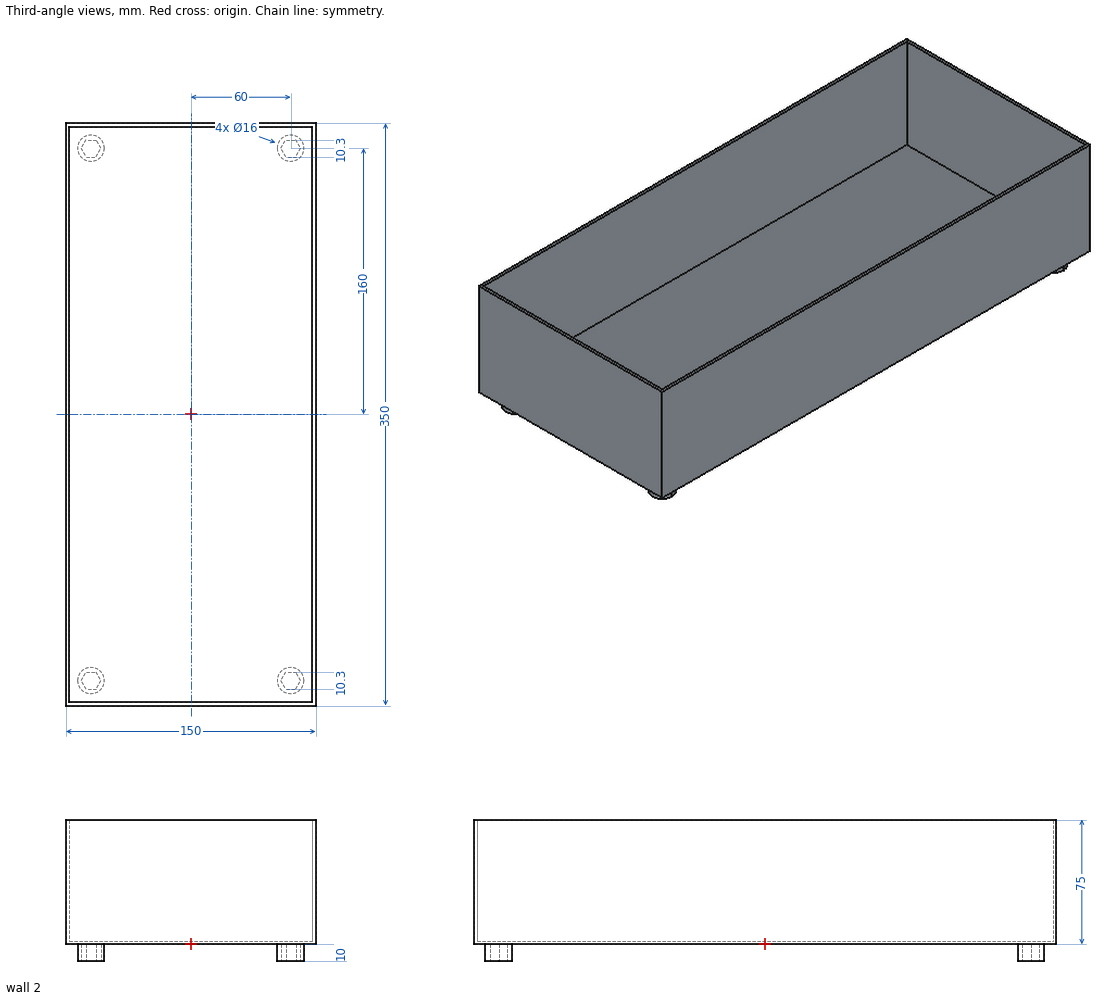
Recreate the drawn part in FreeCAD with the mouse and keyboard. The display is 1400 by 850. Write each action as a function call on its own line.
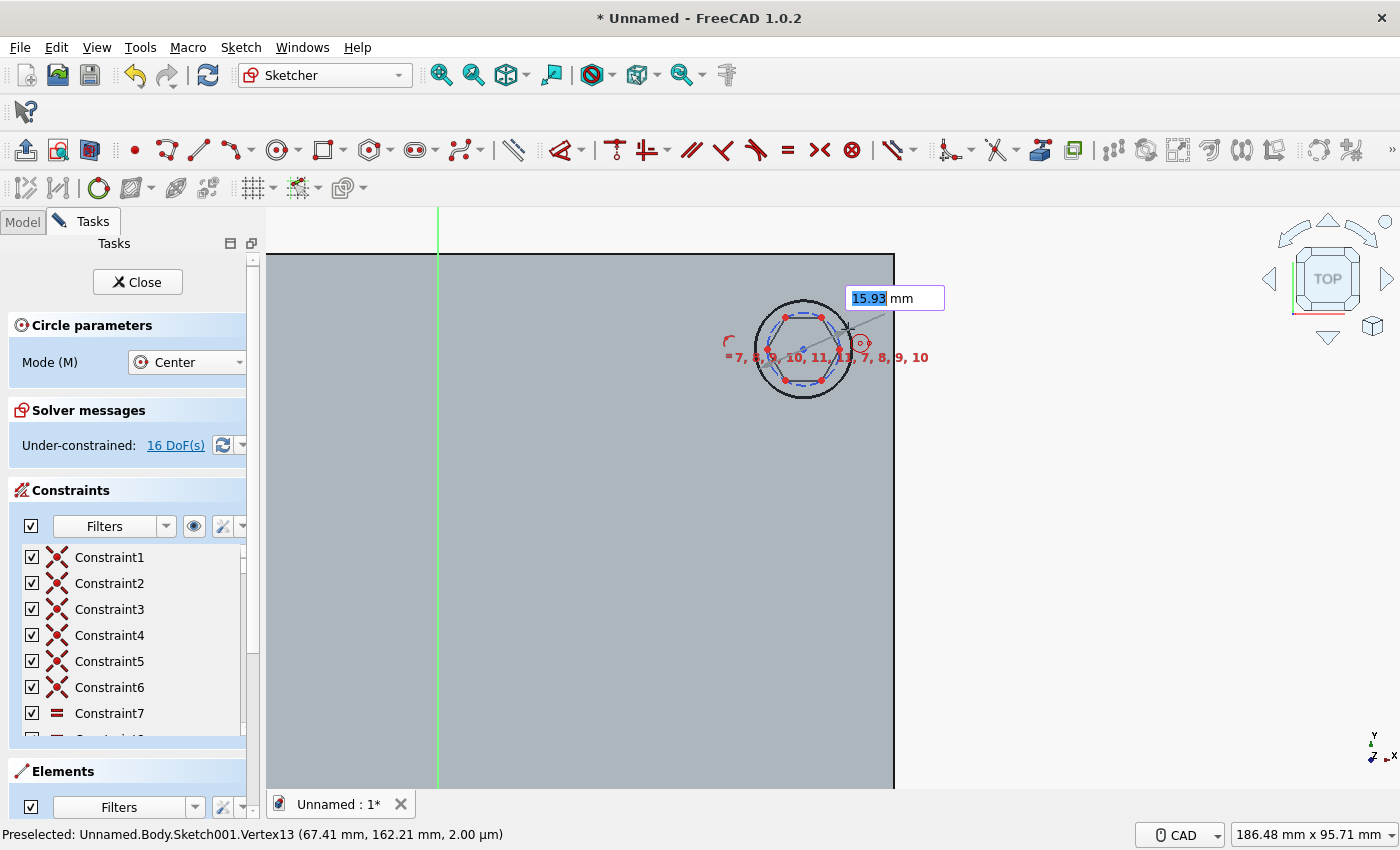
text(16)
key(Return)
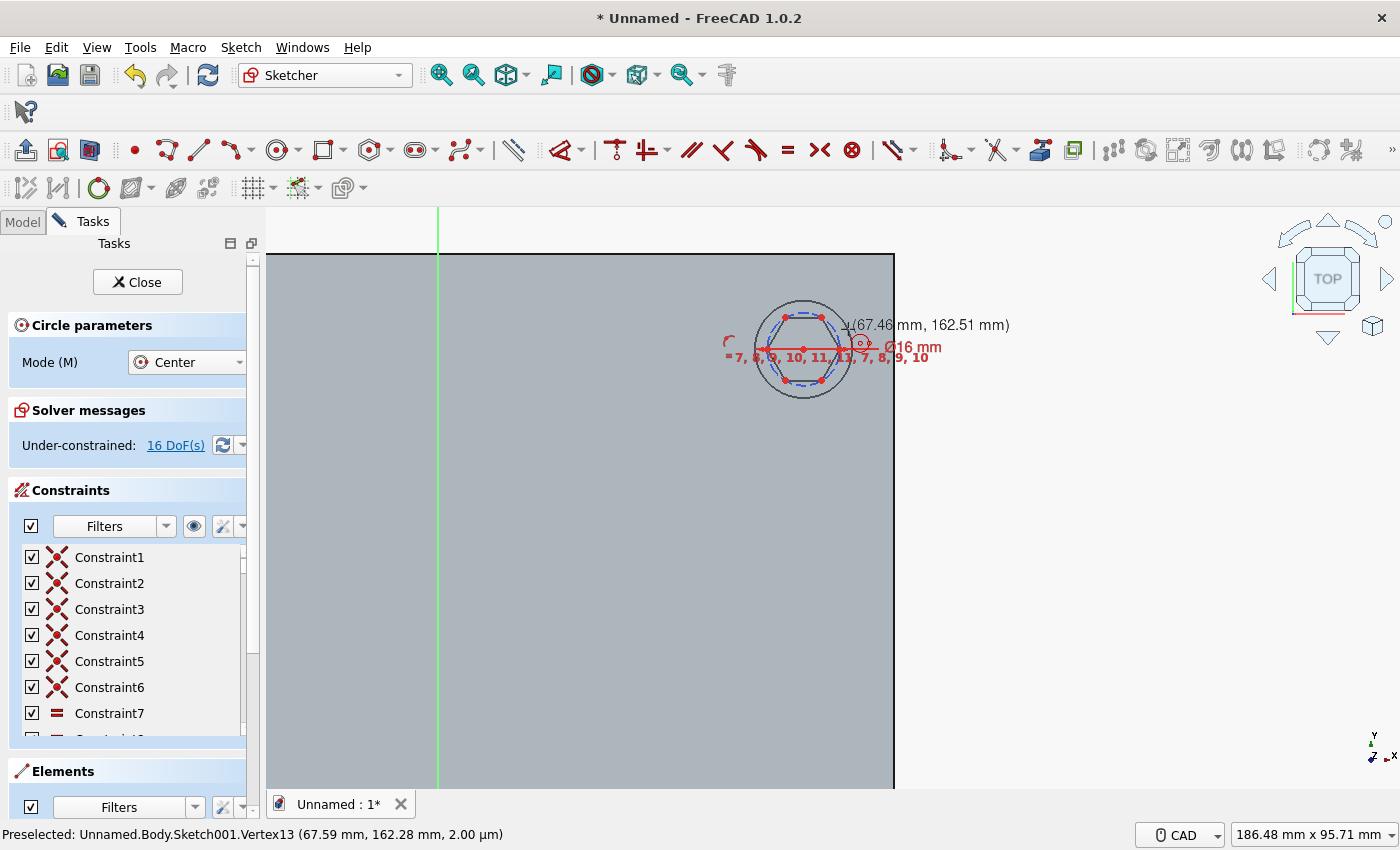
scroll(829, 336, down, 9)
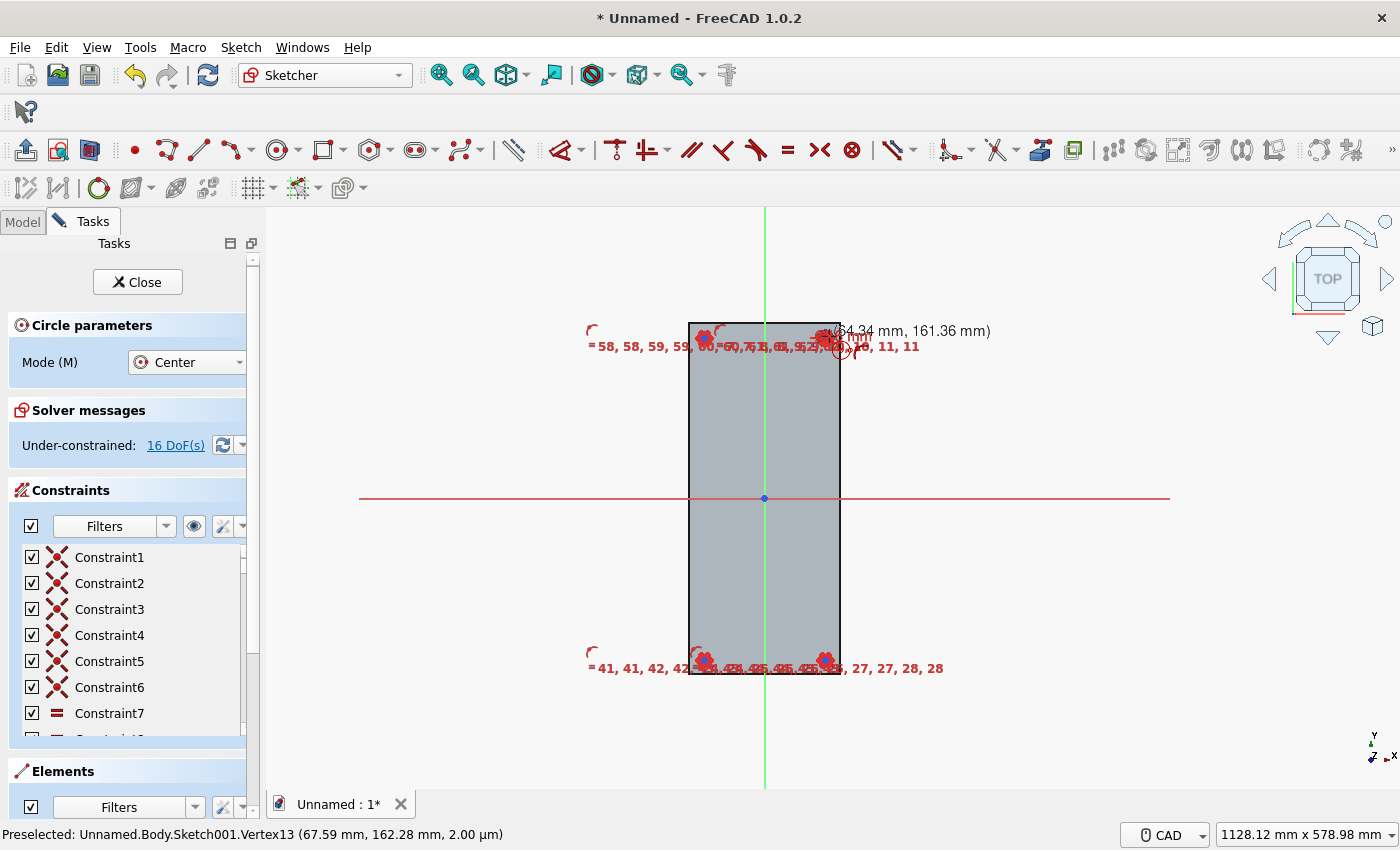
scroll(825, 659, up, 6)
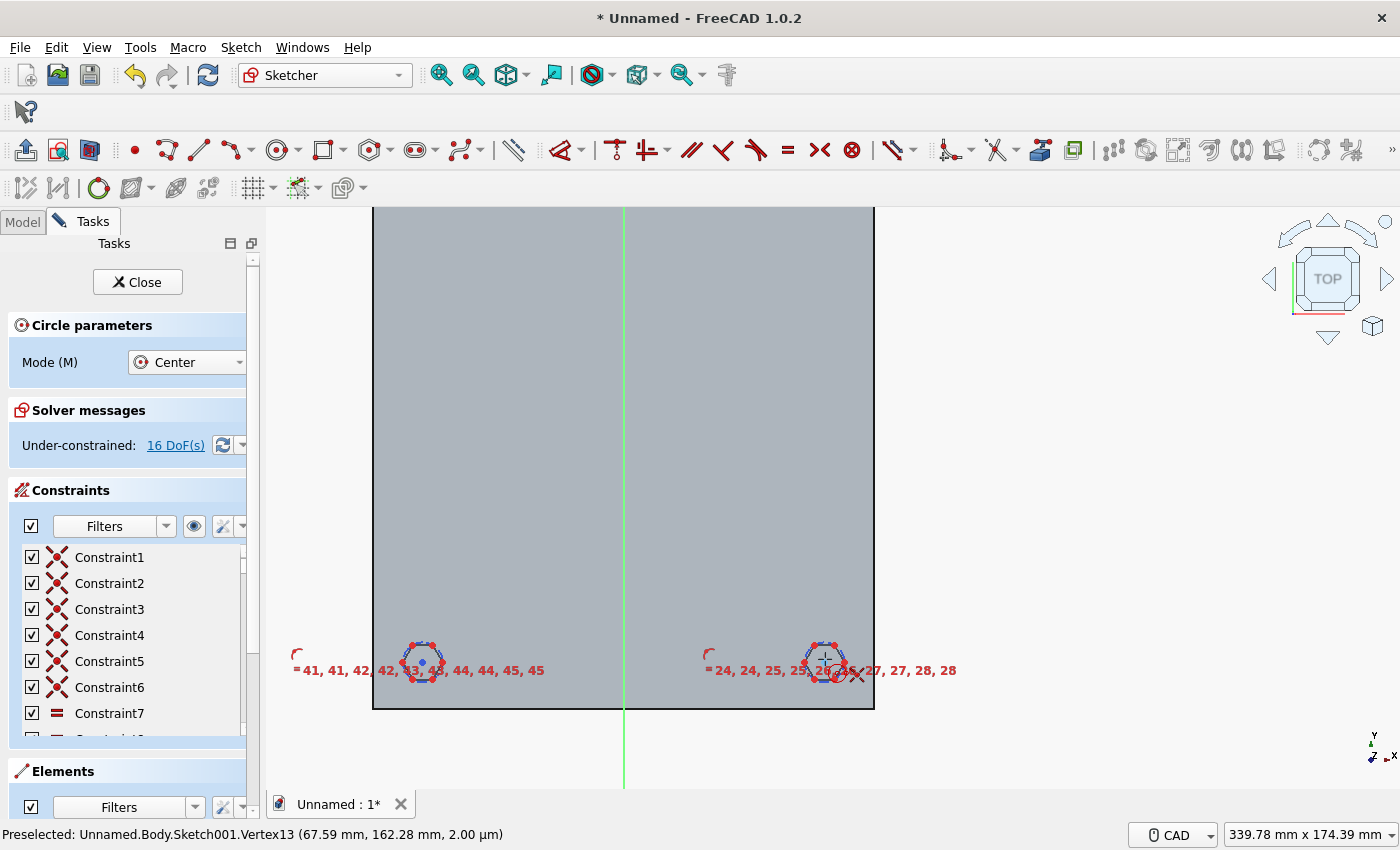
click(825, 662)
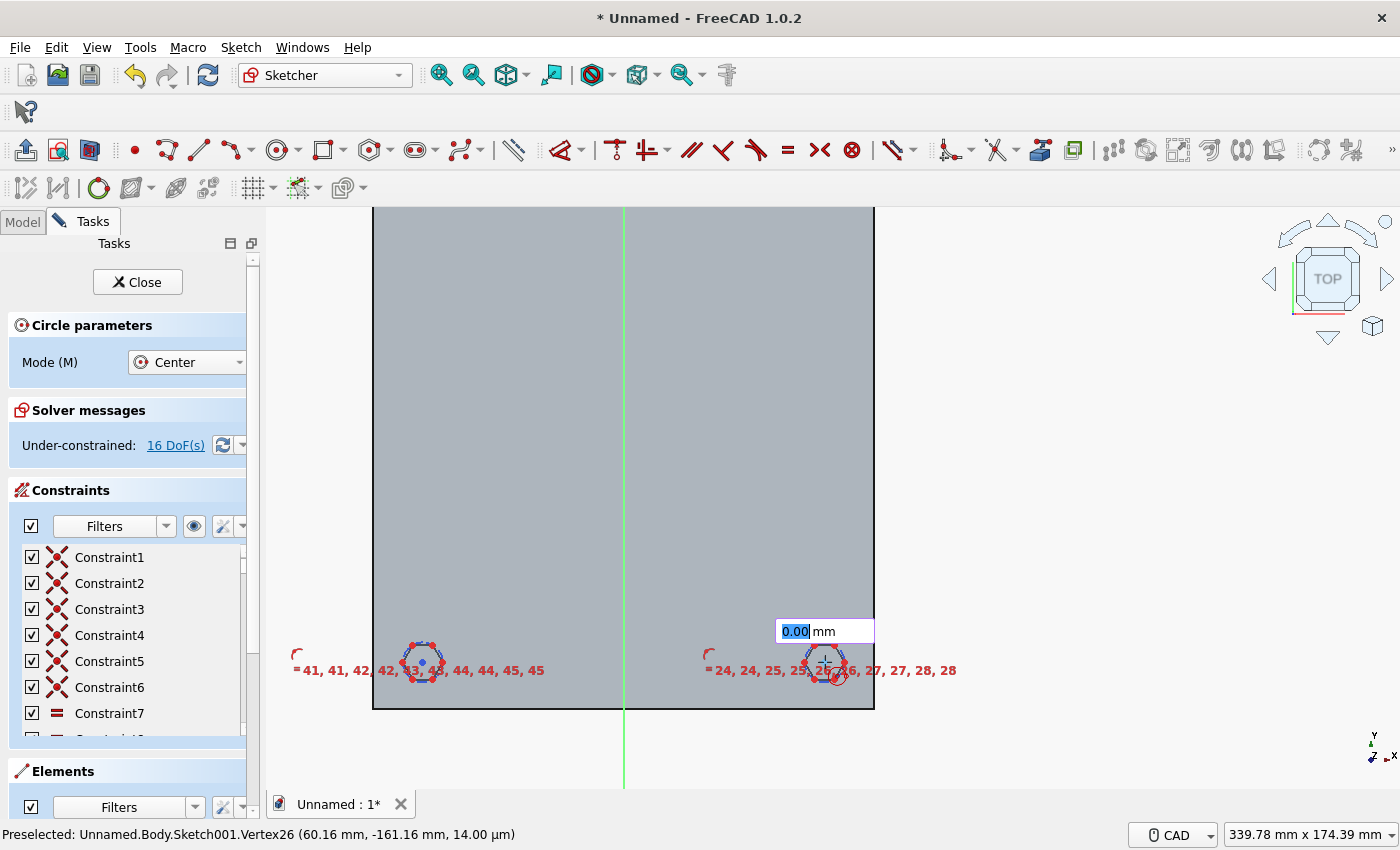
scroll(849, 649, up, 3)
move(849, 649)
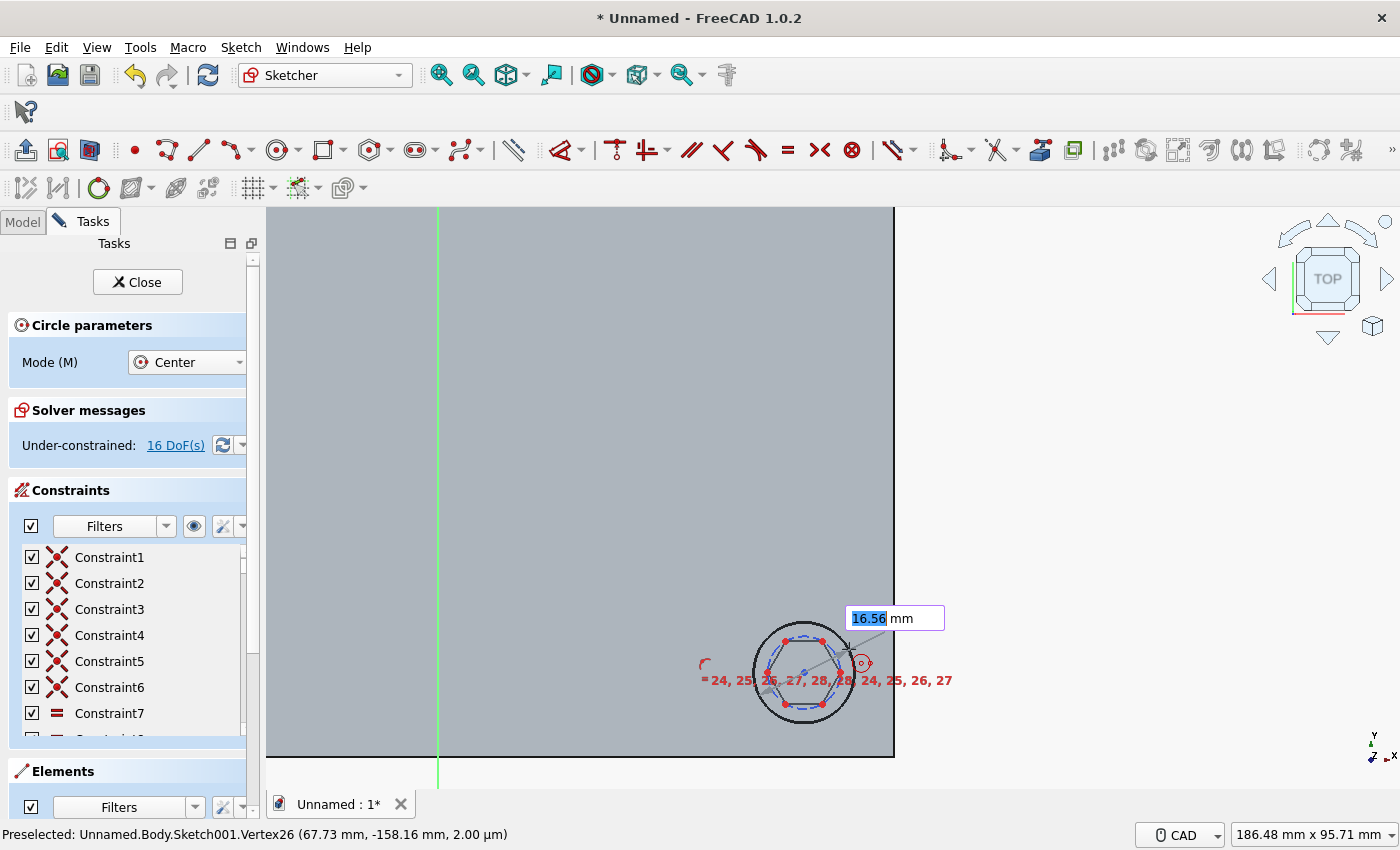
text(16)
key(Return)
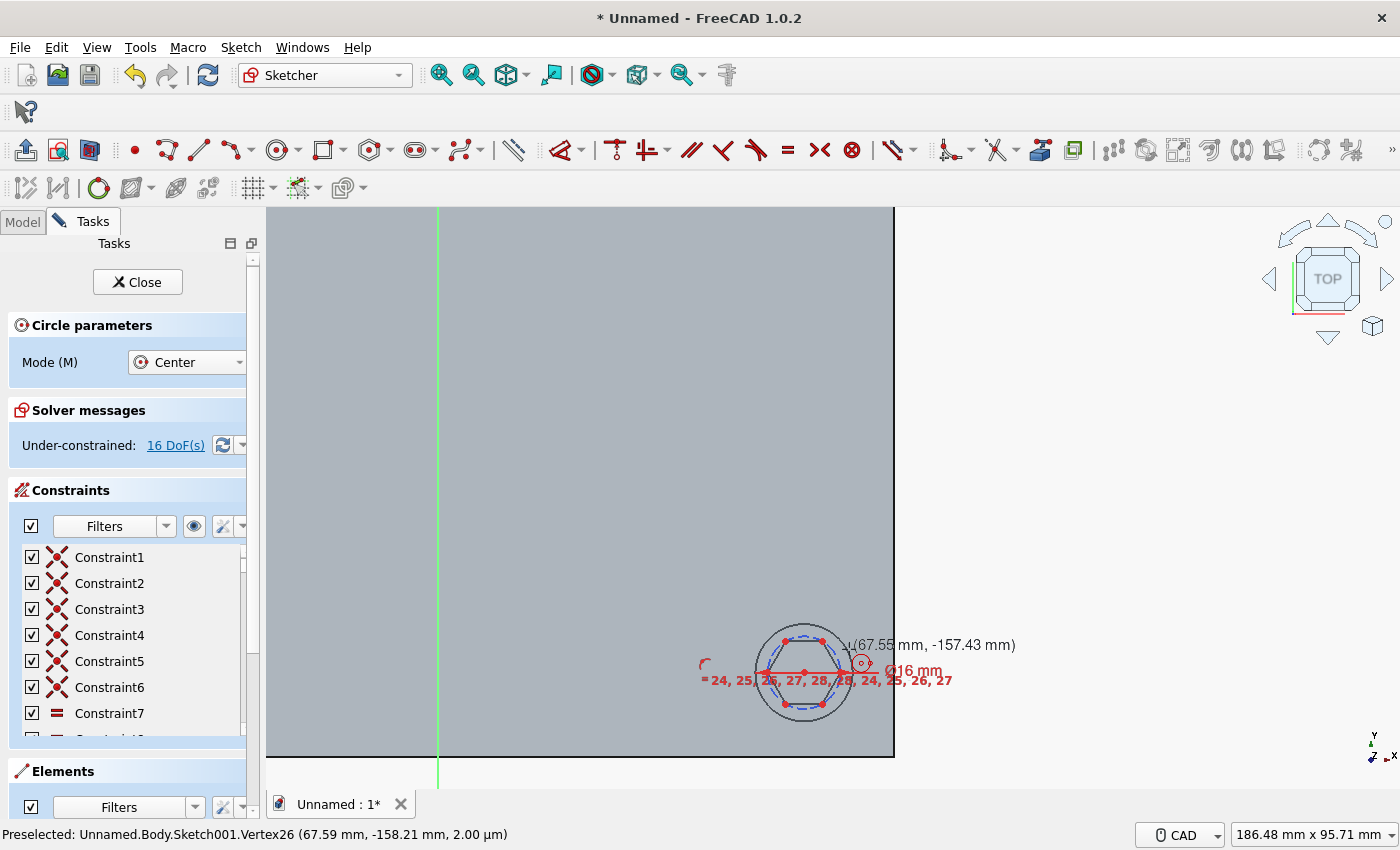
scroll(829, 657, down, 9)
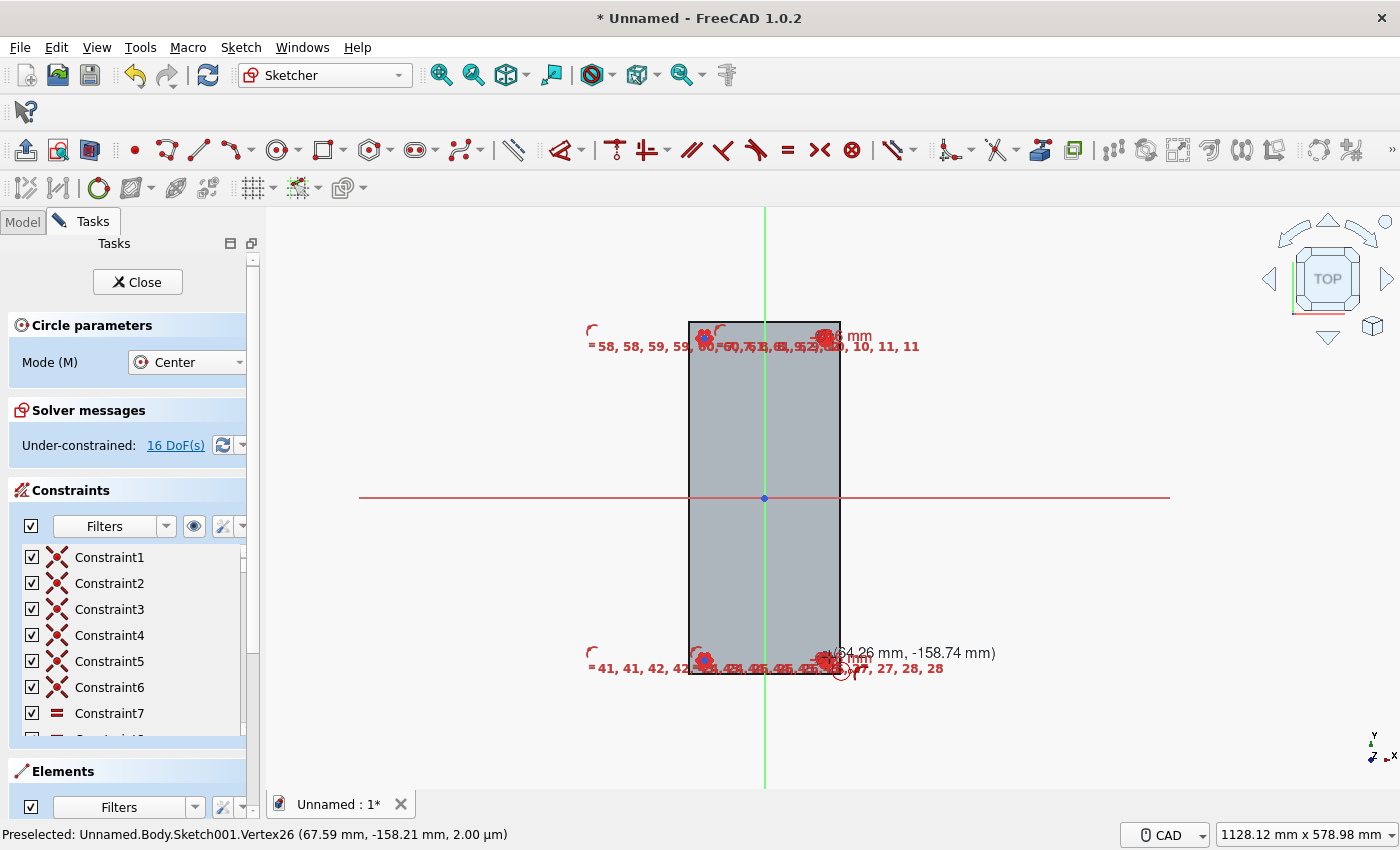
scroll(705, 659, up, 6)